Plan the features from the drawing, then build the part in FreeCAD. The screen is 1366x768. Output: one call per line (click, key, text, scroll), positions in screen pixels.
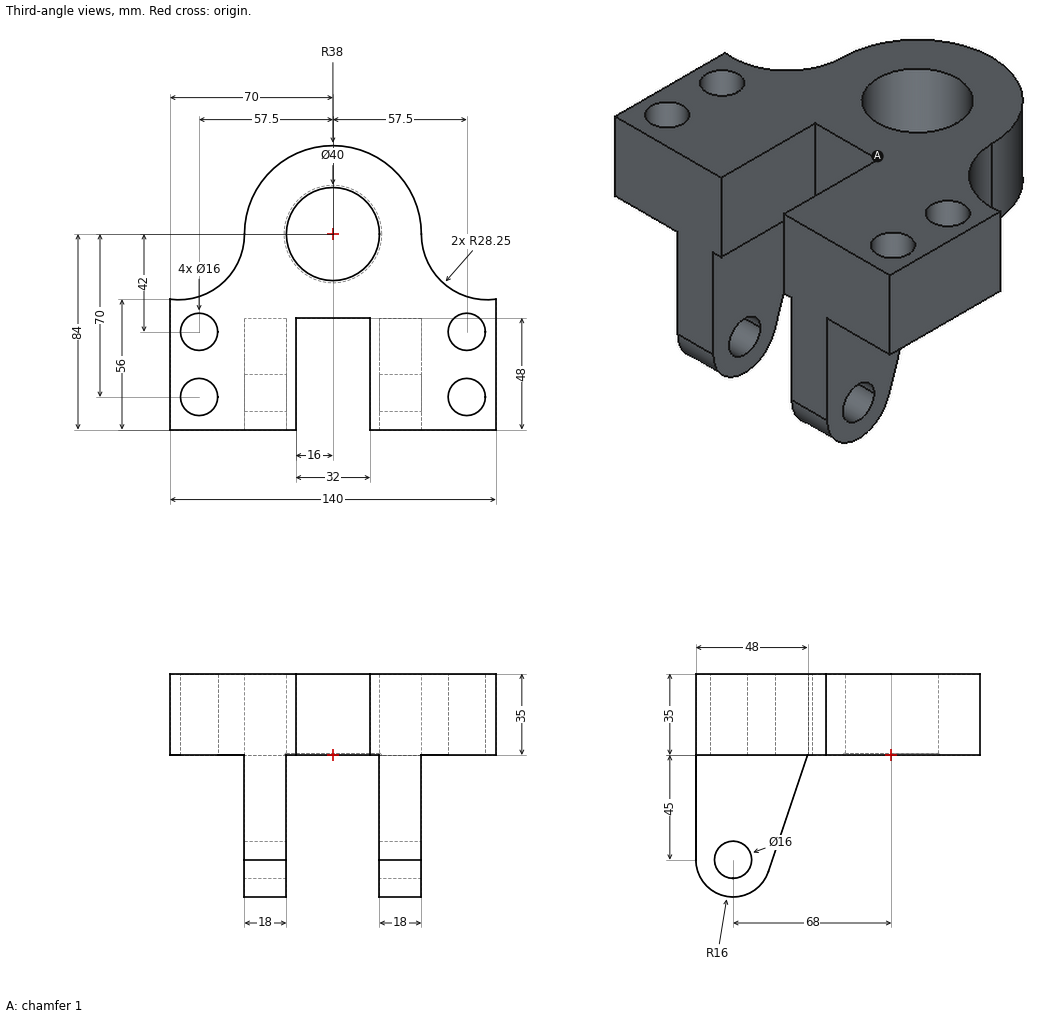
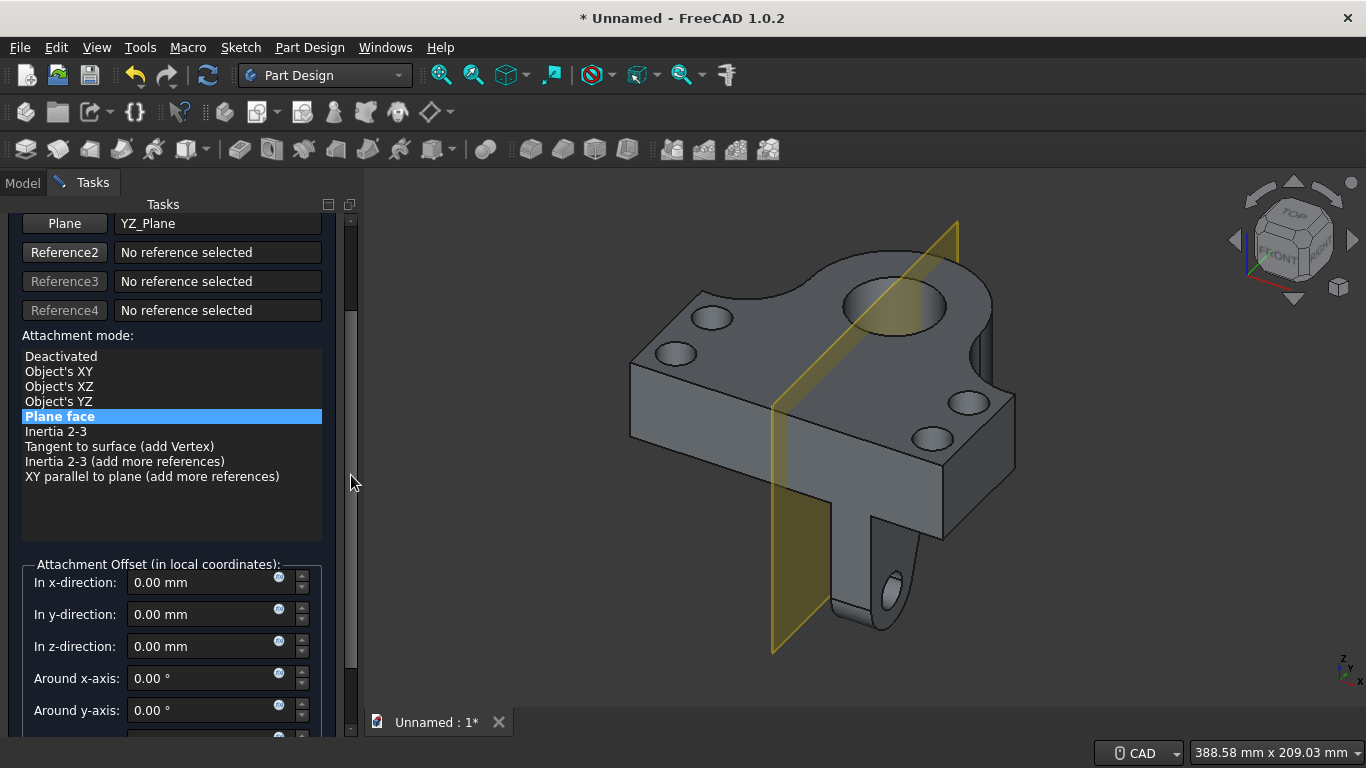
triple_click(210, 646)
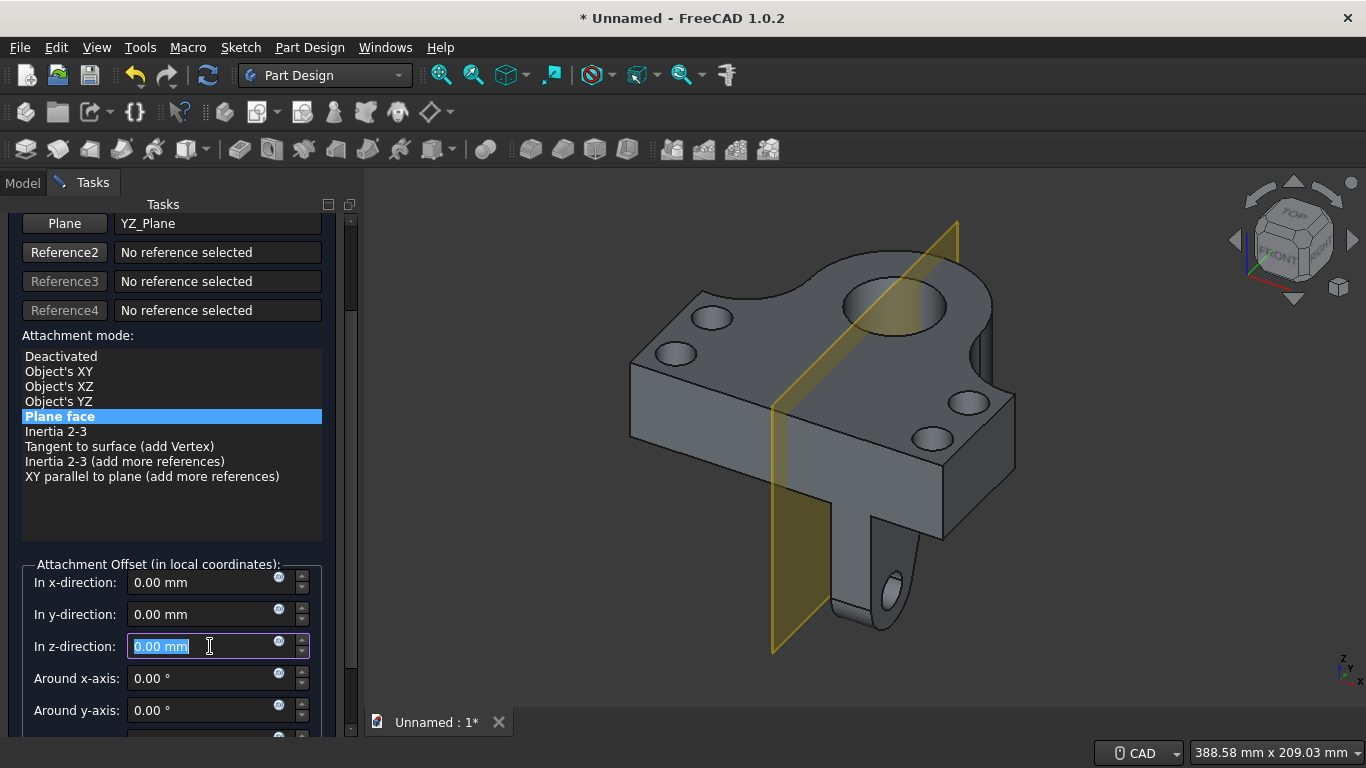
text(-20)
key(Tab)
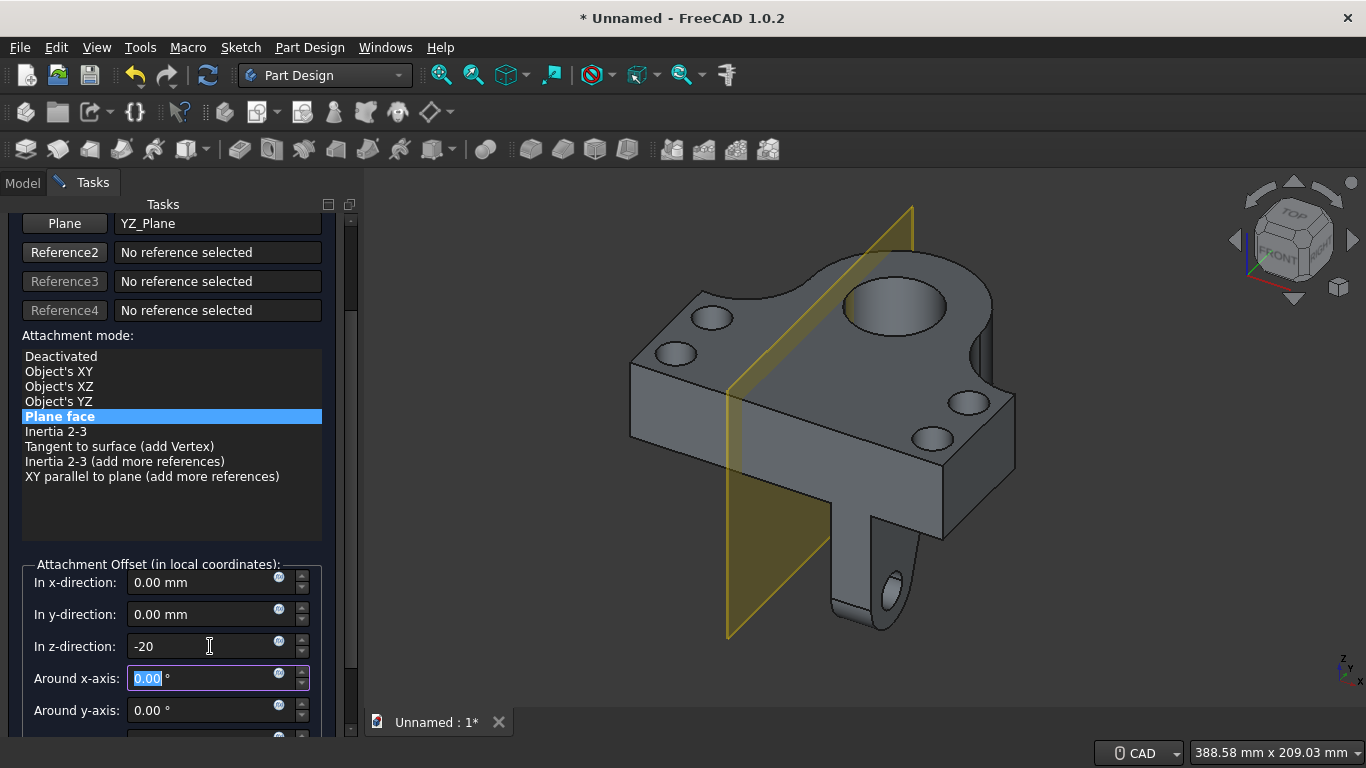
scroll(351, 475, up, 3)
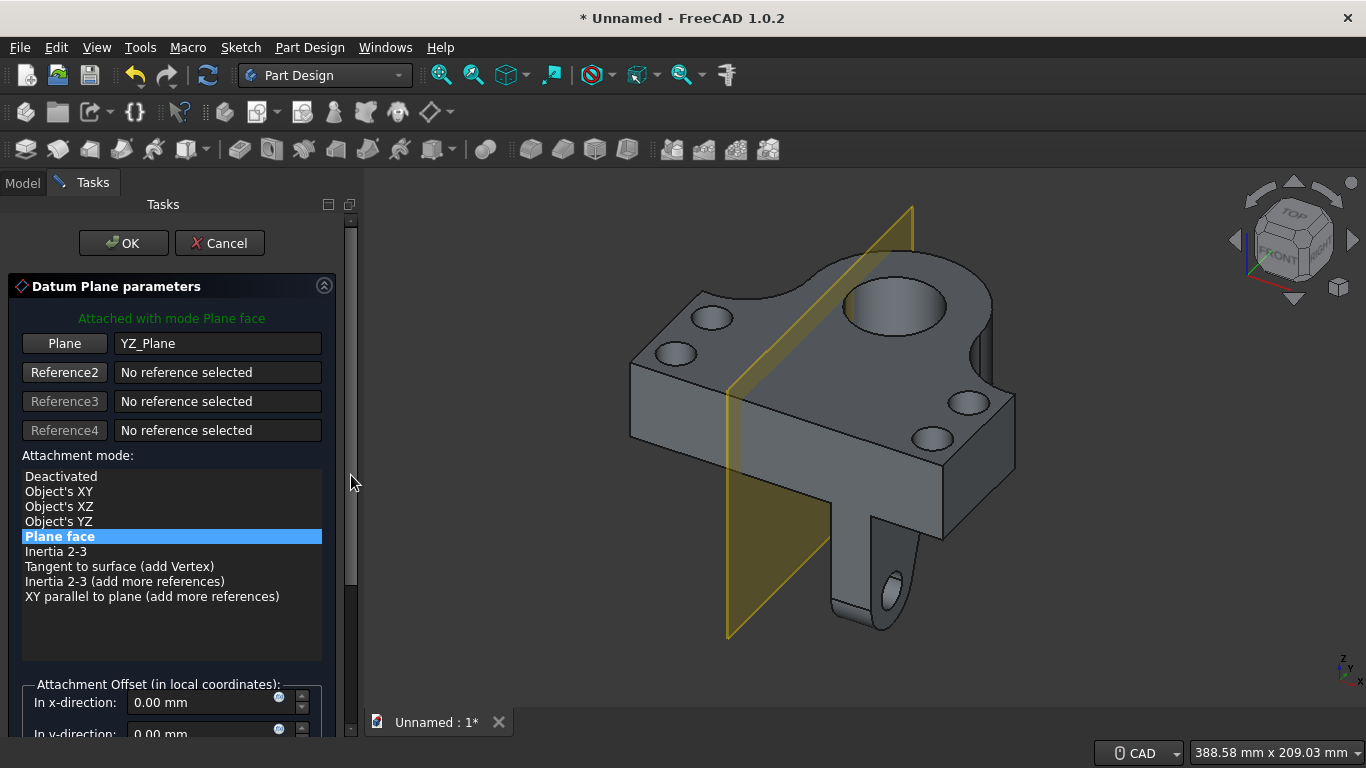
click(124, 243)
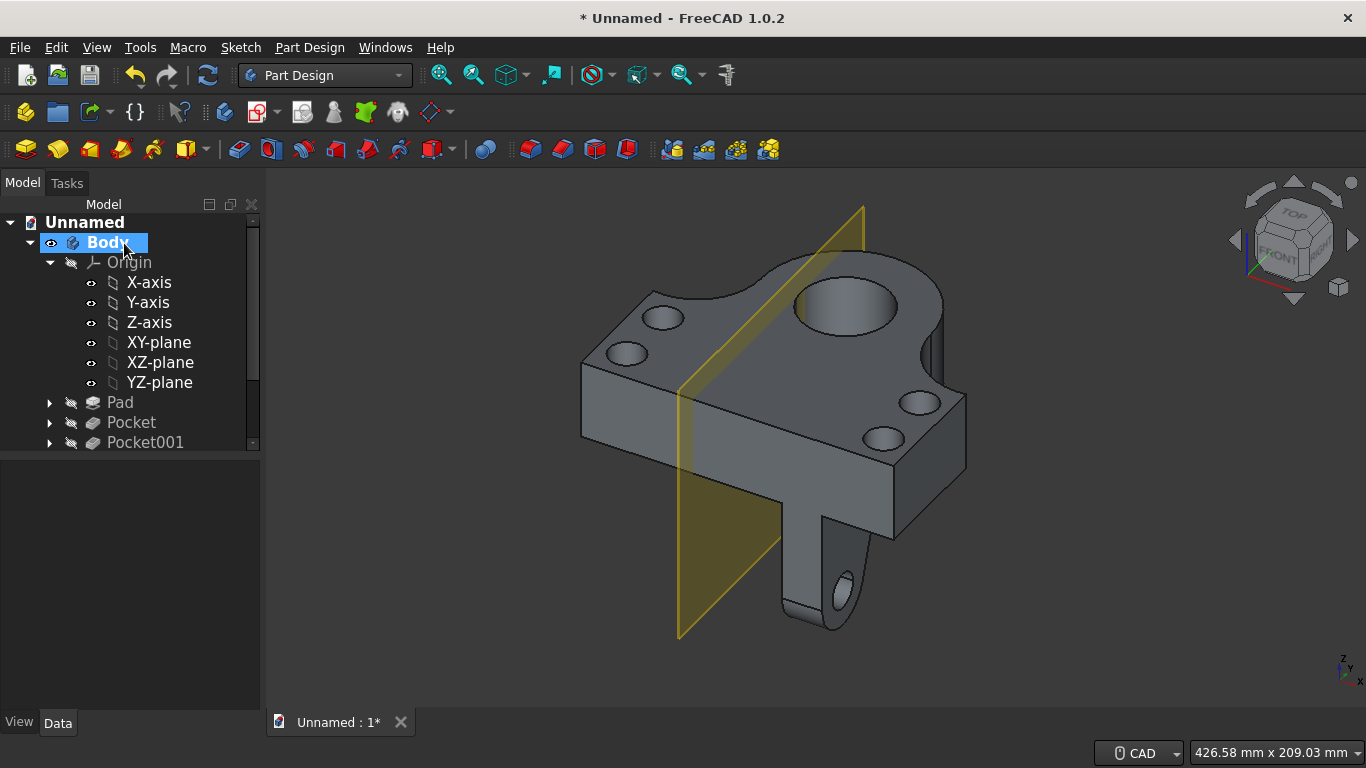
scroll(100, 338, down, 3)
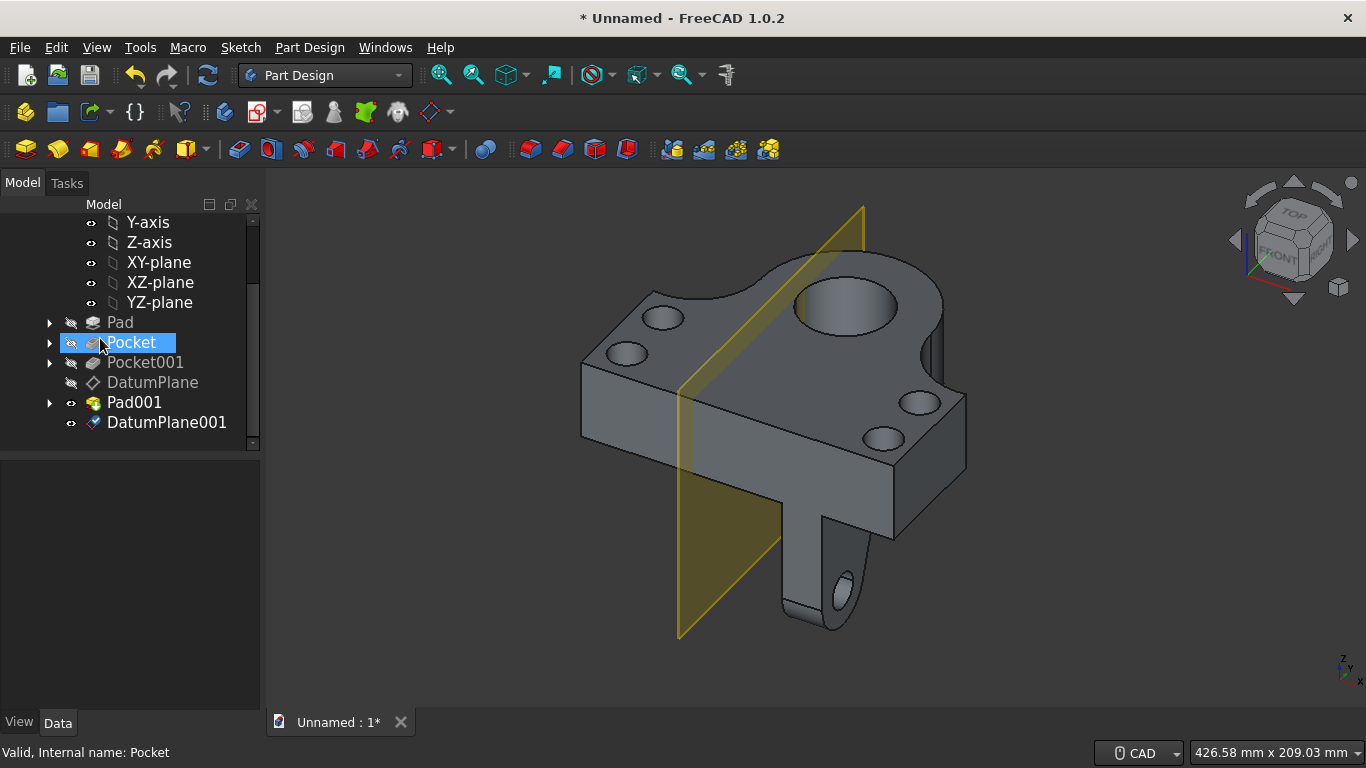
click(116, 423)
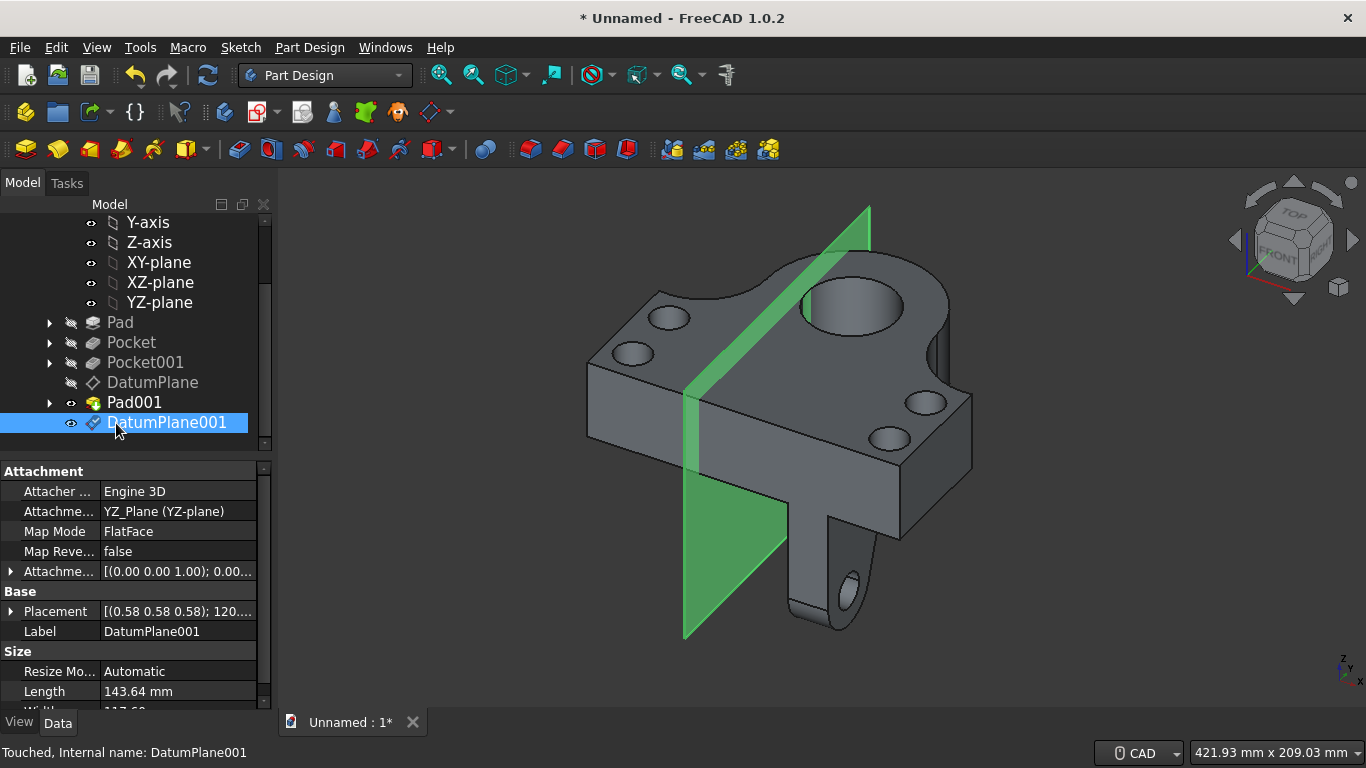
click(258, 112)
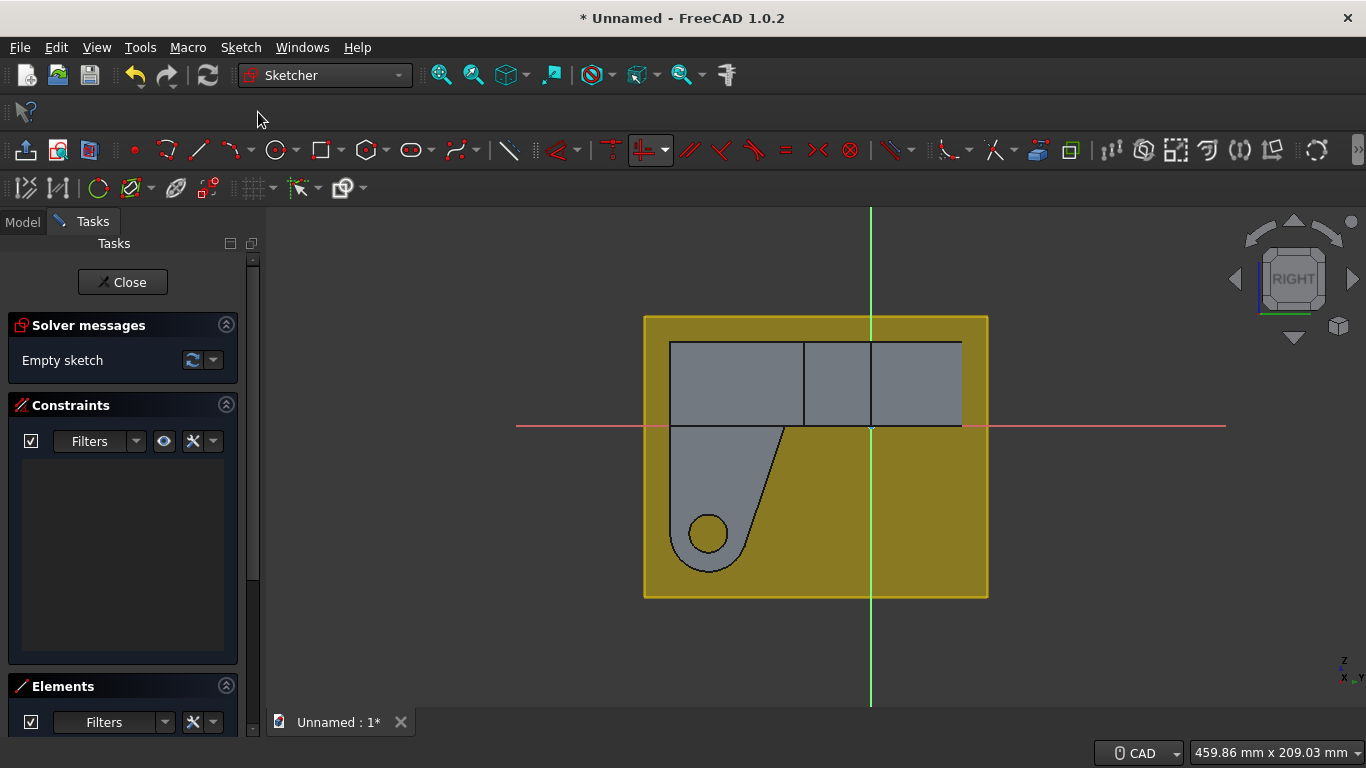
key(q)
key(s)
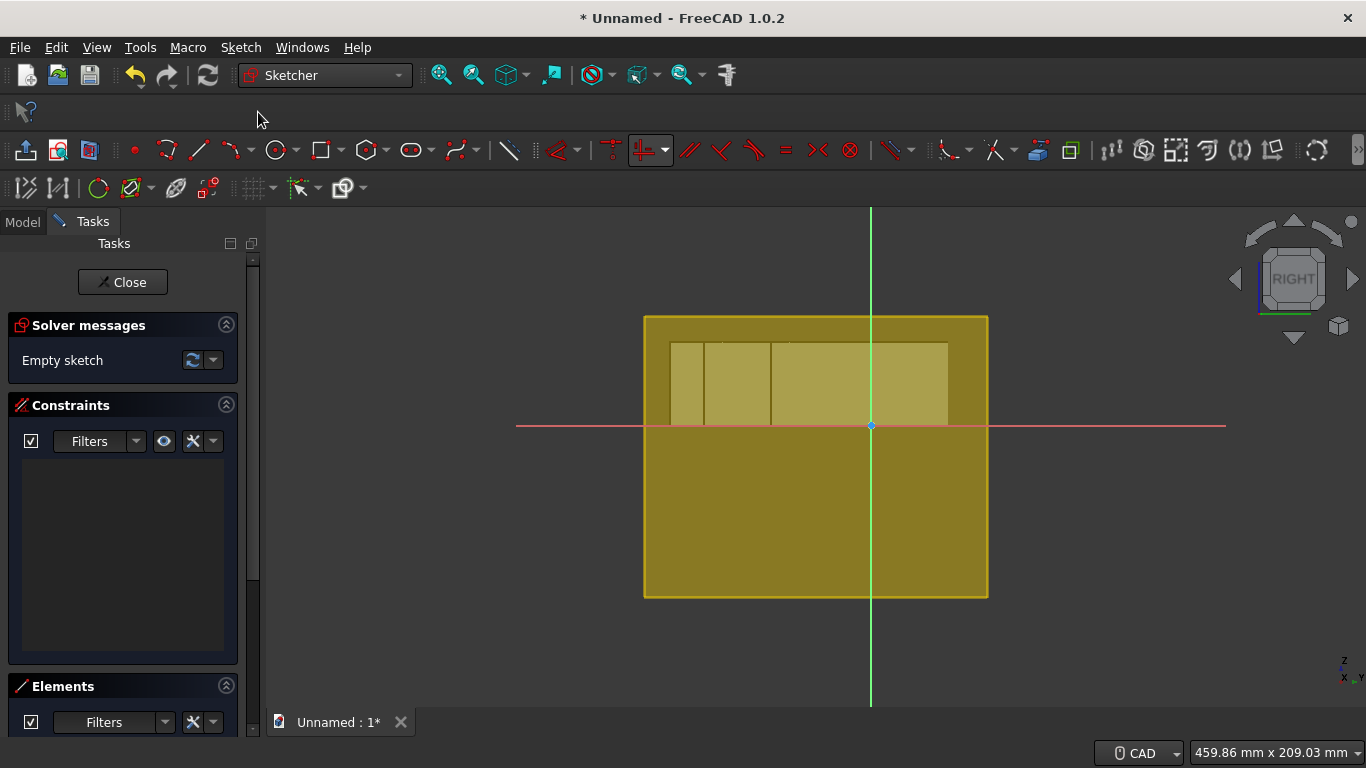
scroll(789, 533, up, 4)